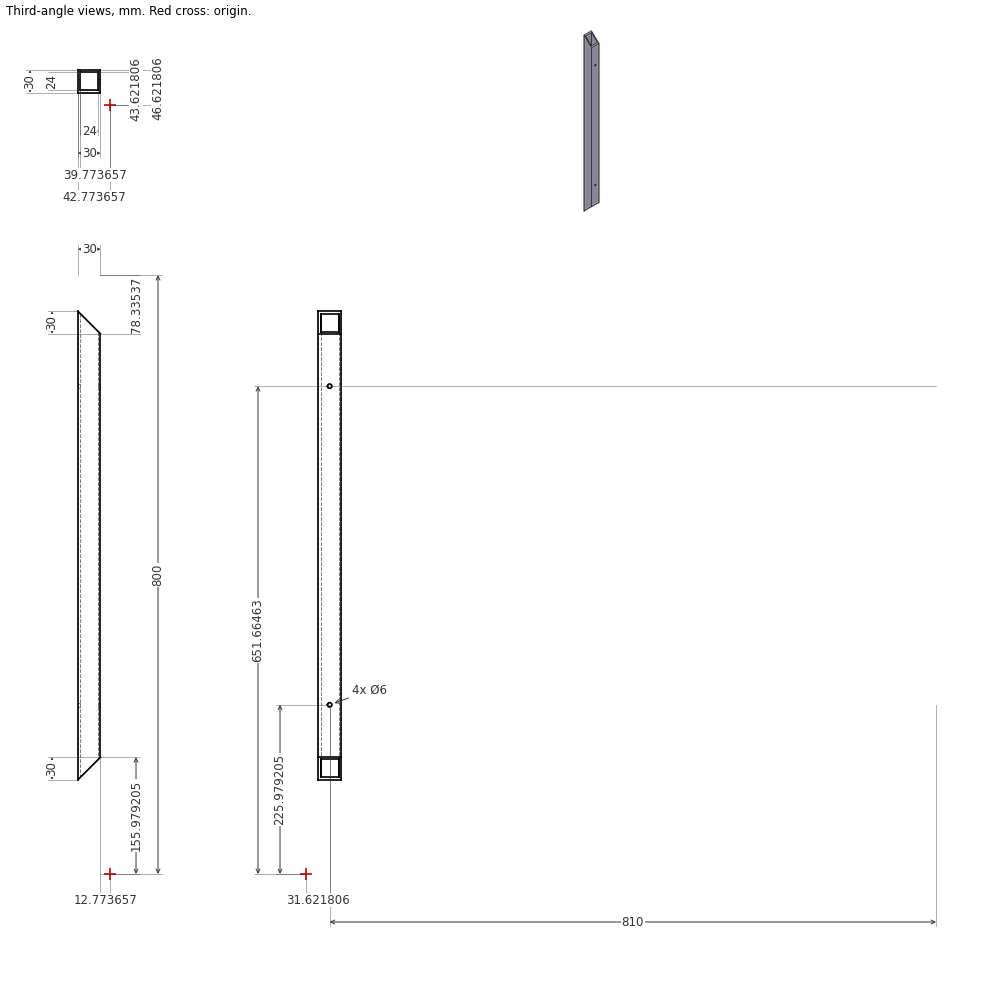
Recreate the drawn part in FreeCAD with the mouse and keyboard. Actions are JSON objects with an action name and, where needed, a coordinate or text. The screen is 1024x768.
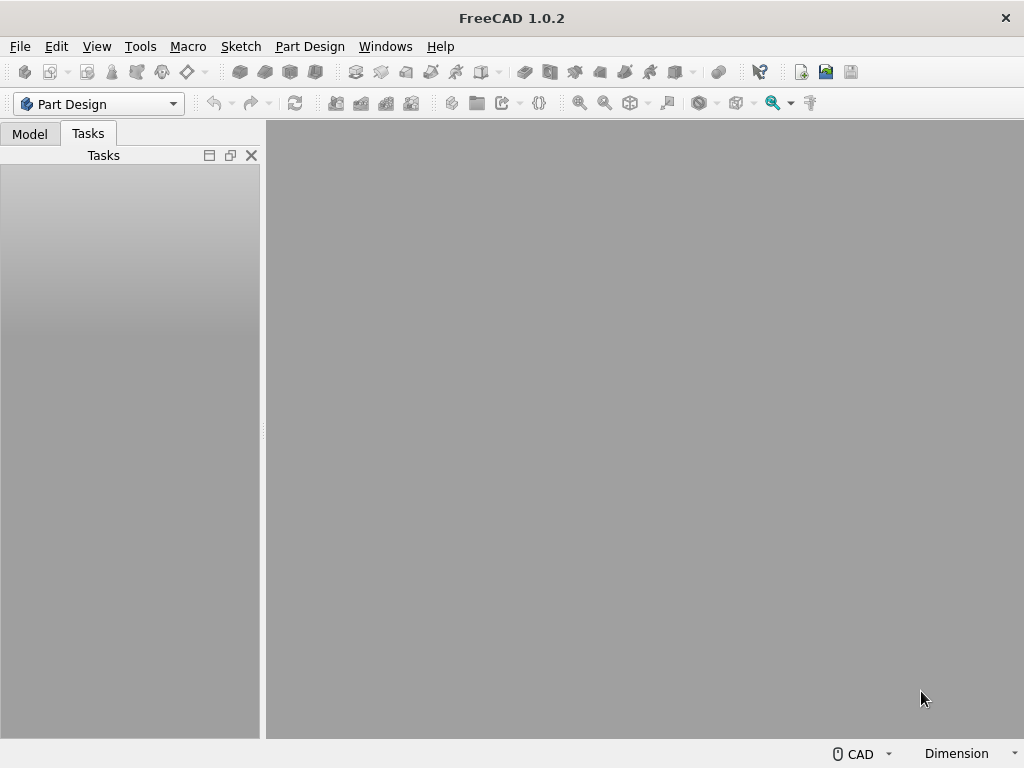
{"action": "key", "text": "ctrl+n"}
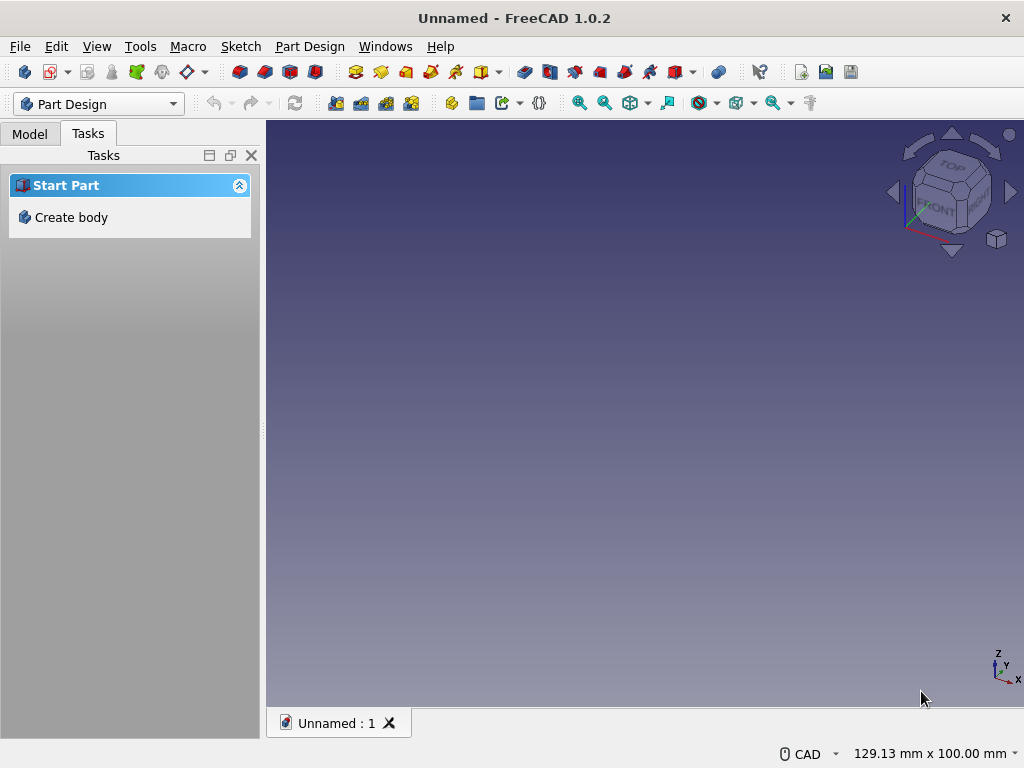
{"action": "left_click", "coordinate": [50, 72]}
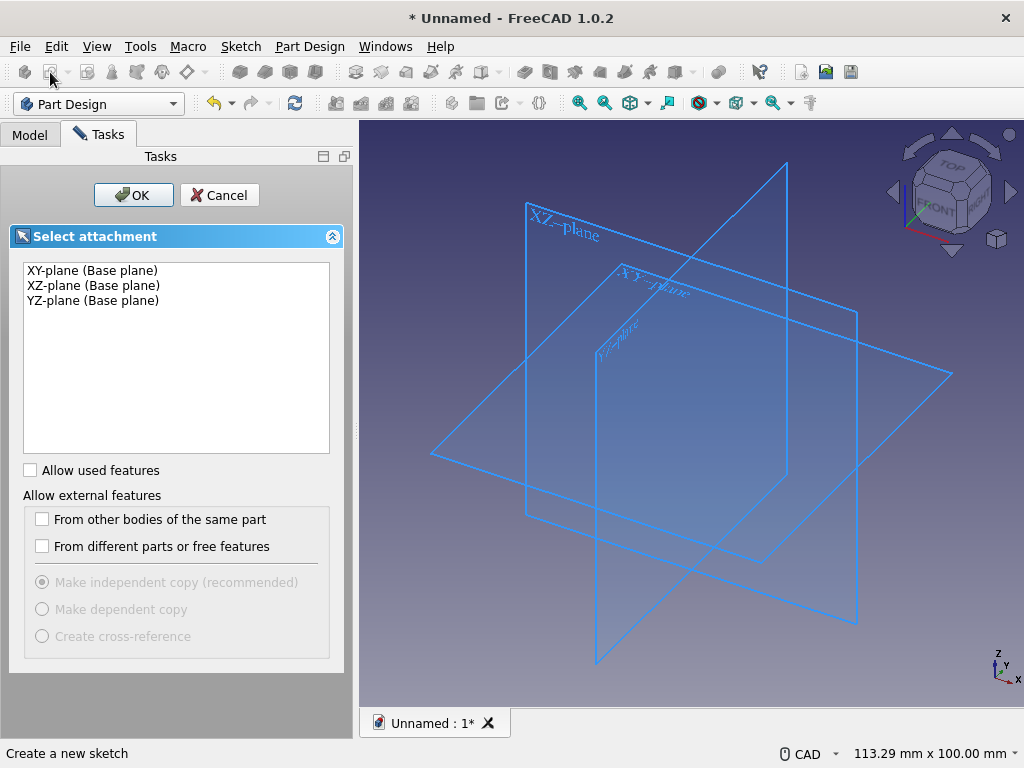
{"action": "left_click", "coordinate": [84, 270]}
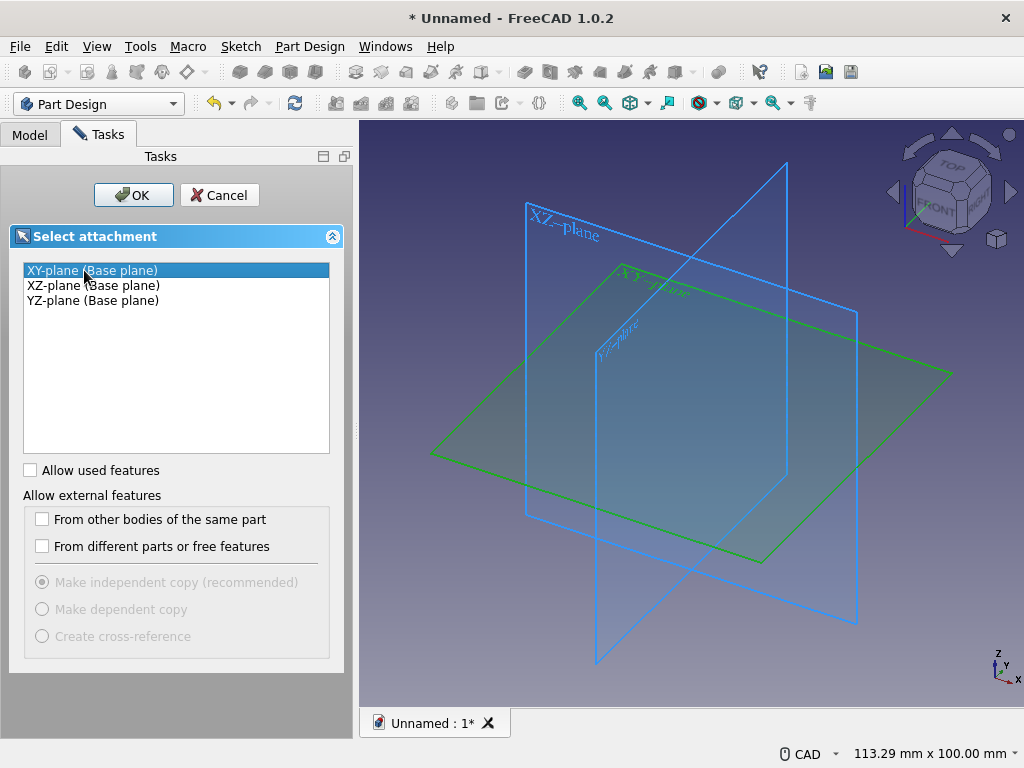
{"action": "left_click", "coordinate": [134, 195]}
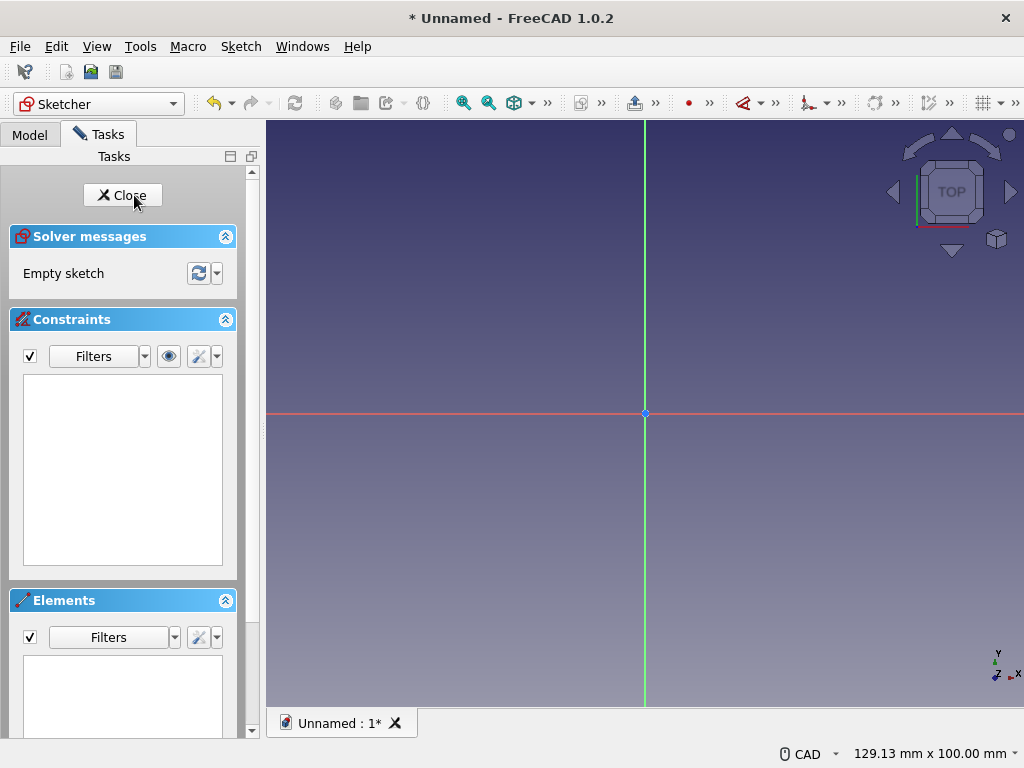
{"action": "scroll", "coordinate": [834, 679], "scroll_direction": "down", "scroll_amount": 1}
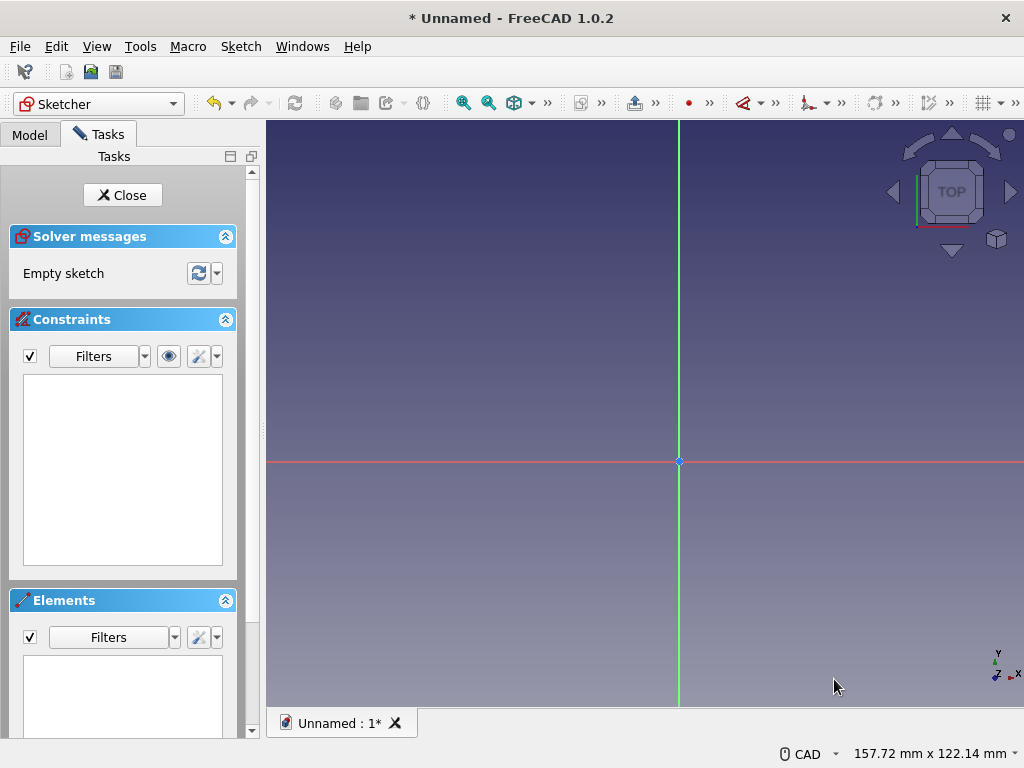
{"action": "scroll", "coordinate": [577, 272], "scroll_direction": "up", "scroll_amount": 3}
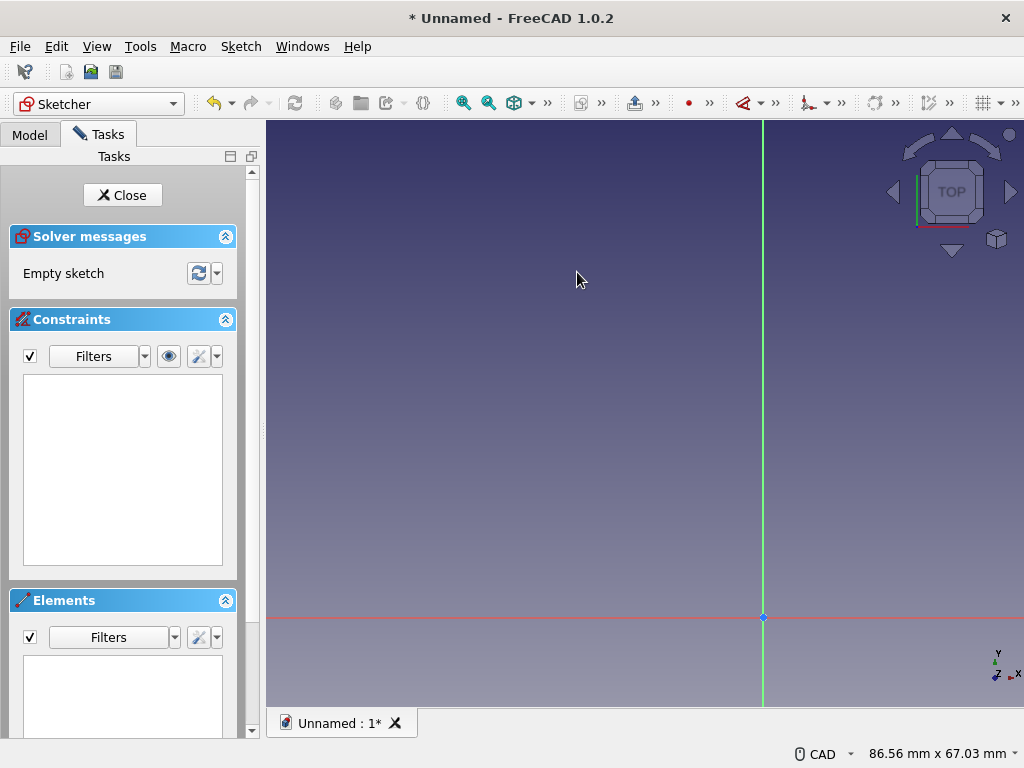
{"action": "key", "text": "g r"}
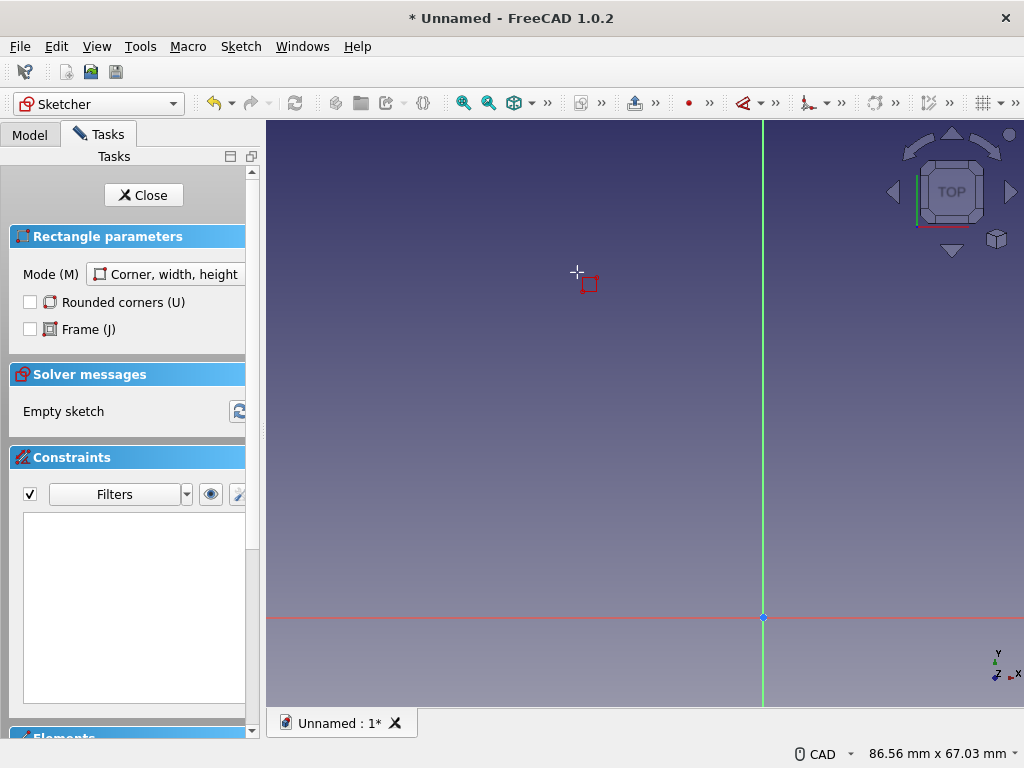
{"action": "left_click", "coordinate": [389, 209]}
{"action": "left_click", "coordinate": [651, 472]}
{"action": "key", "text": "Escape"}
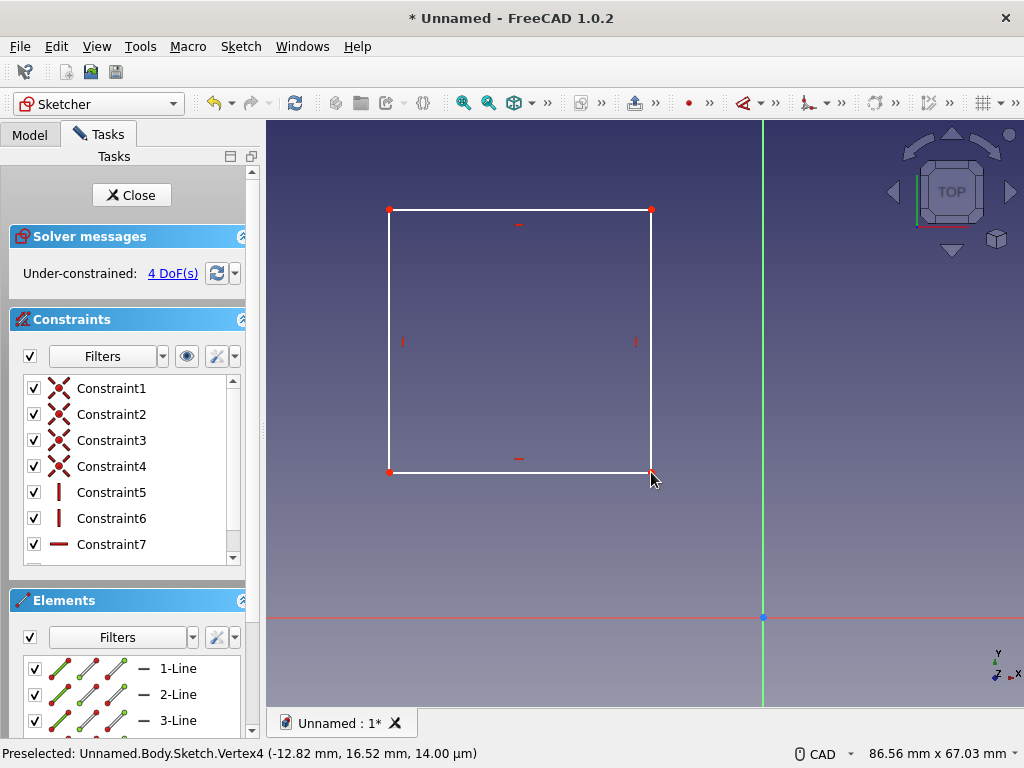
{"action": "key", "text": "d"}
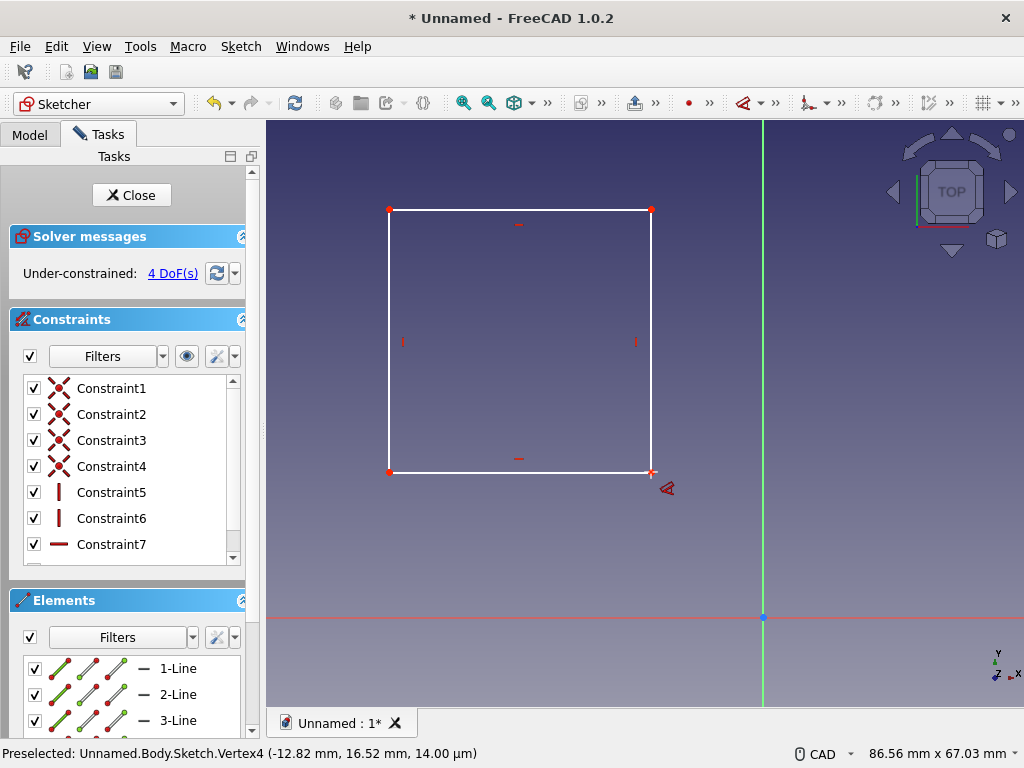
{"action": "left_click", "coordinate": [389, 289]}
{"action": "left_click", "coordinate": [355, 342]}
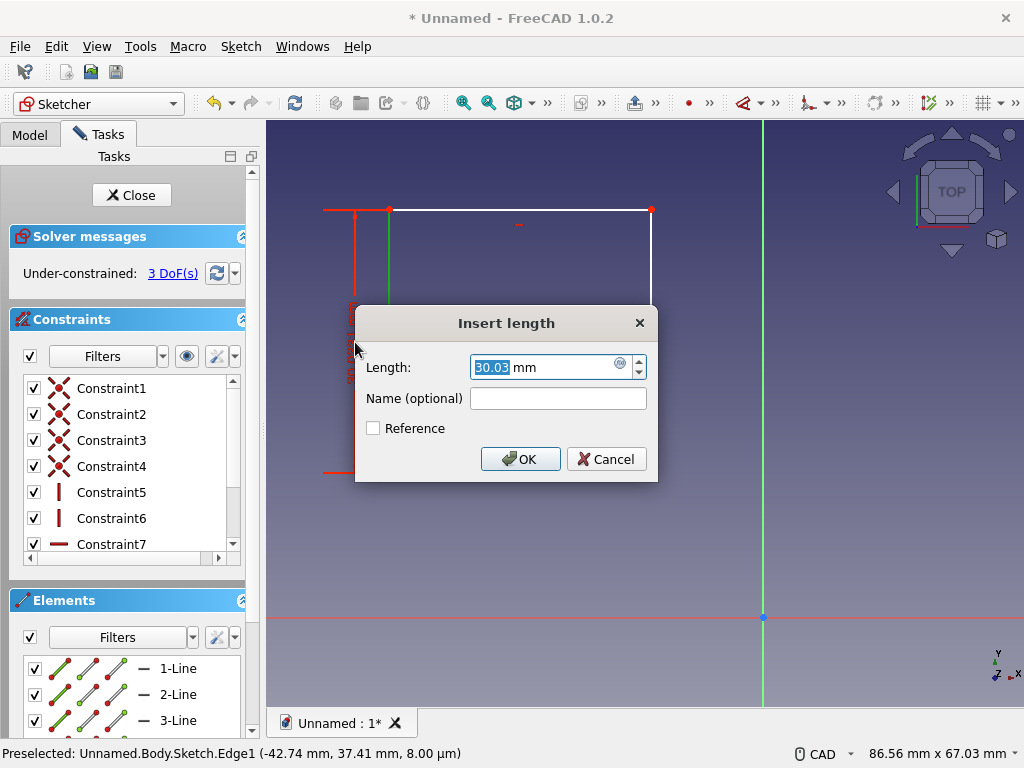
{"action": "type", "text": "30"}
{"action": "key", "text": "Return"}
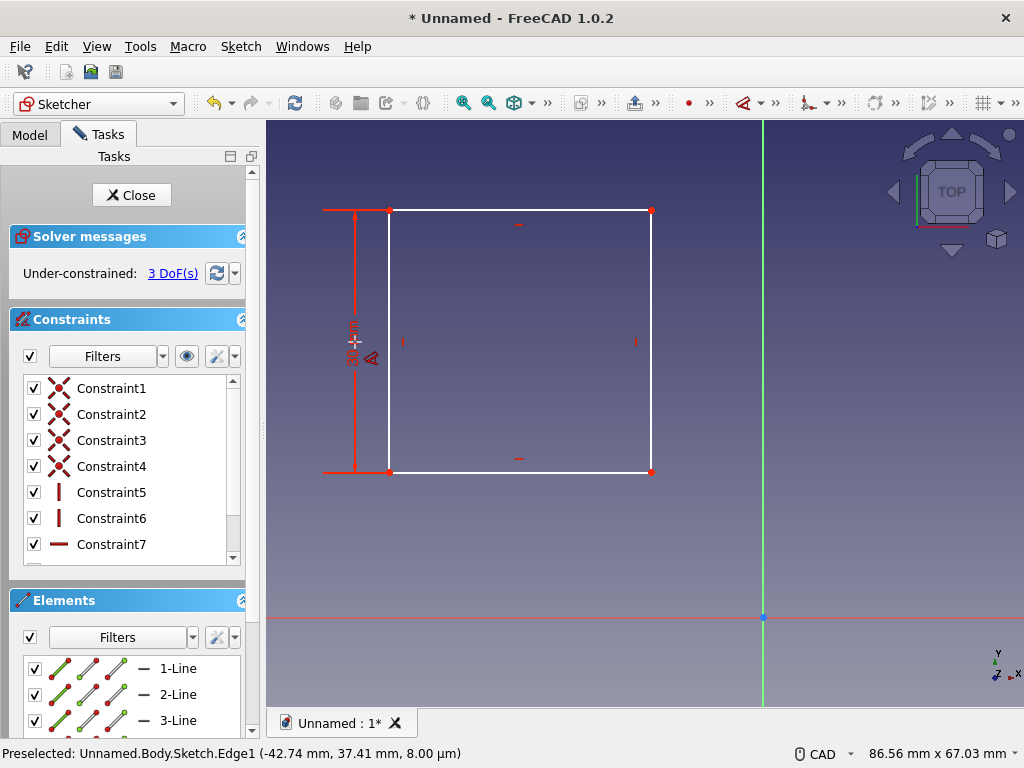
{"action": "left_click", "coordinate": [468, 473]}
{"action": "left_click", "coordinate": [520, 507]}